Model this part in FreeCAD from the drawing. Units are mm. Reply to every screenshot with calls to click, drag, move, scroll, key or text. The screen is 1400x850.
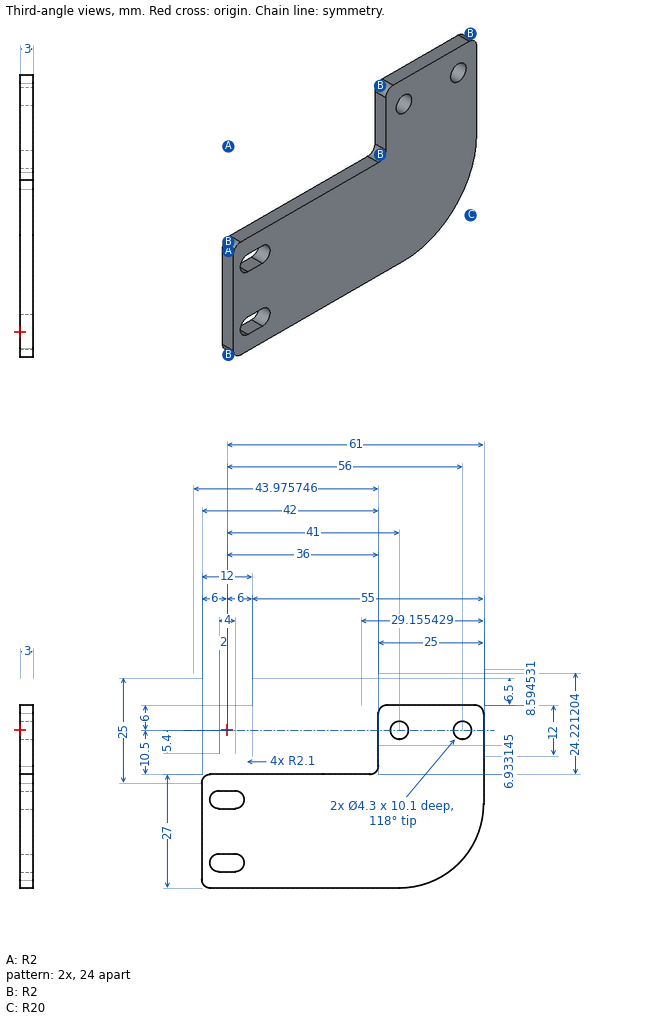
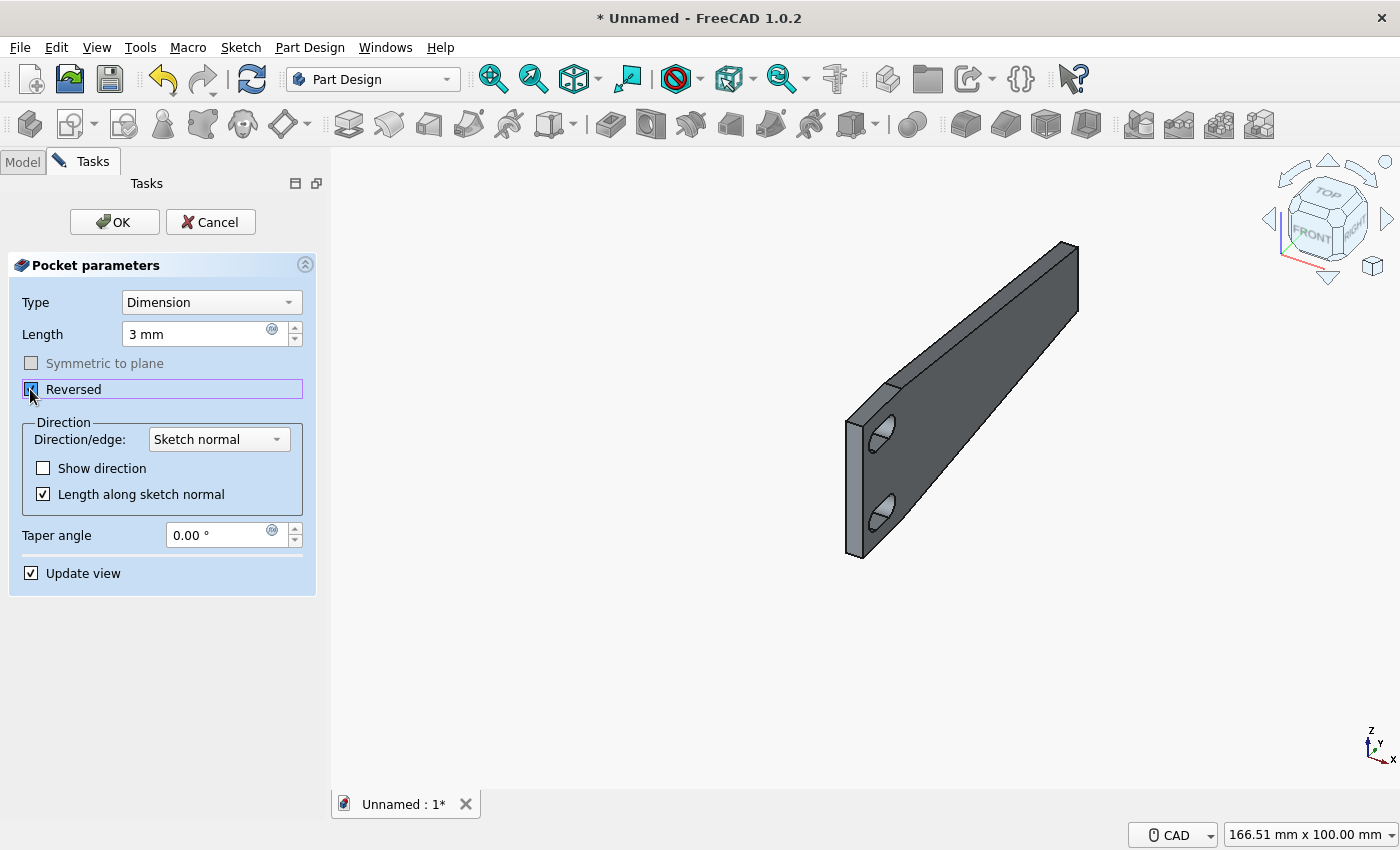
click(115, 222)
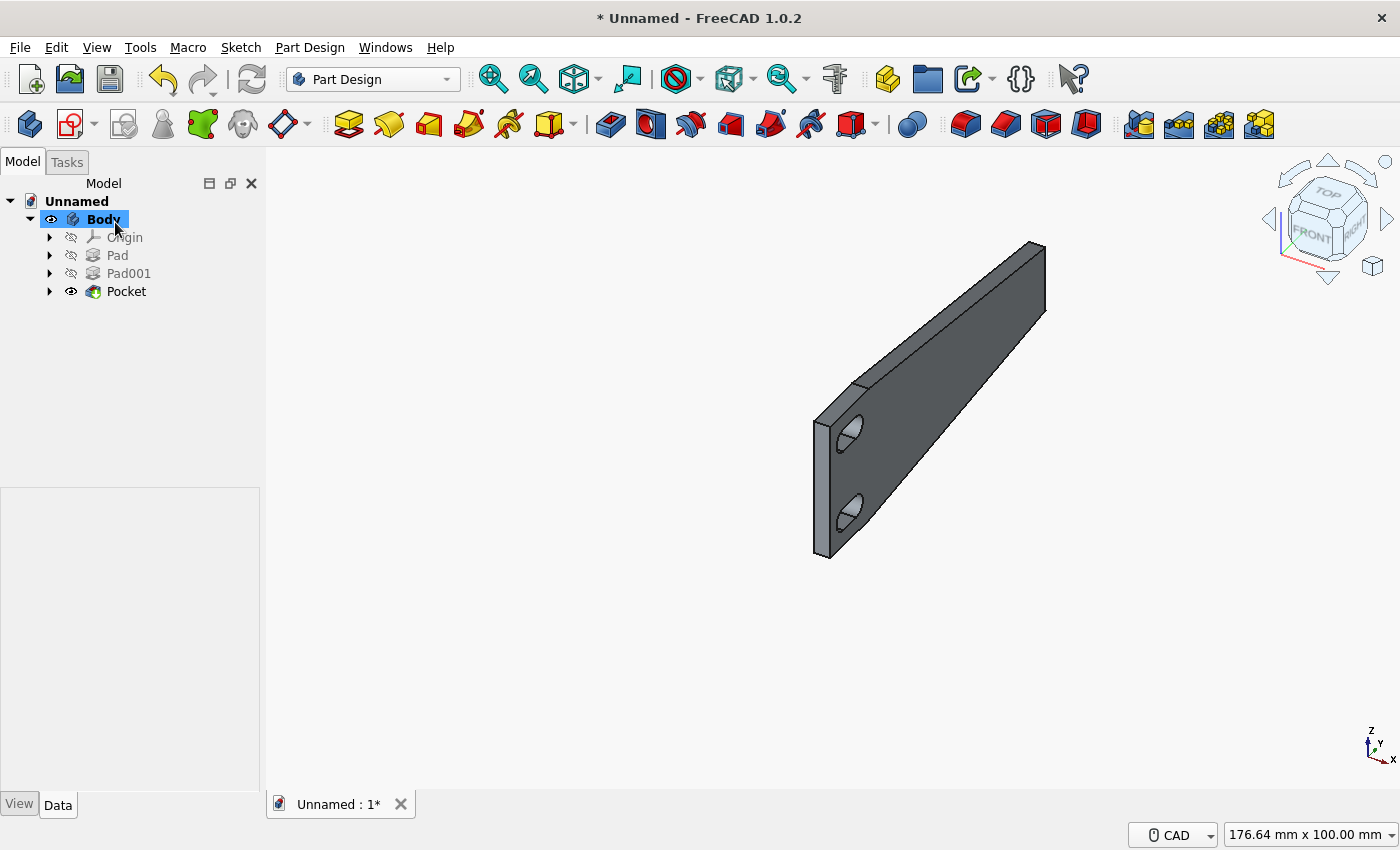
click(822, 423)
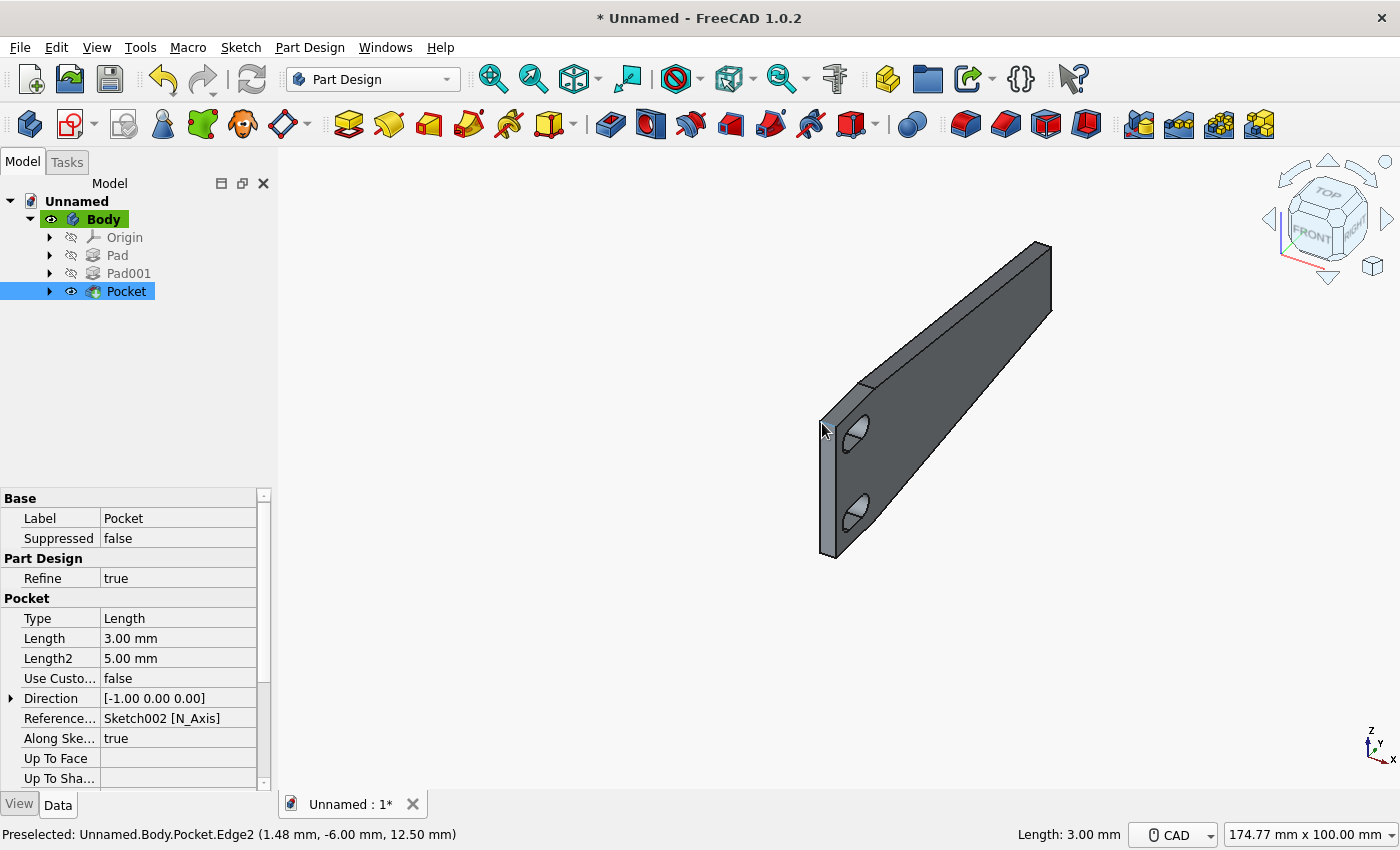
scroll(828, 555, up, 4)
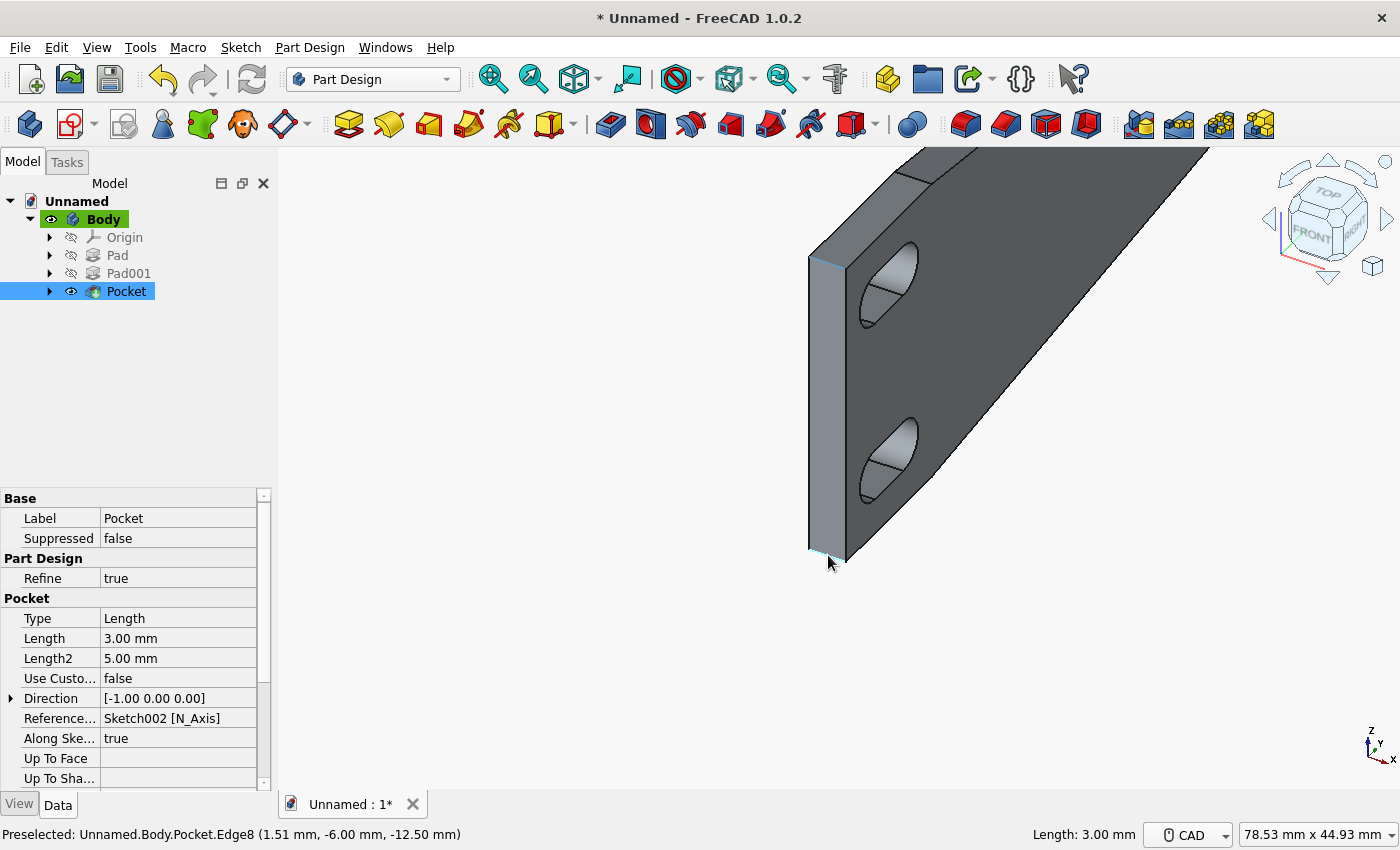
click(494, 80)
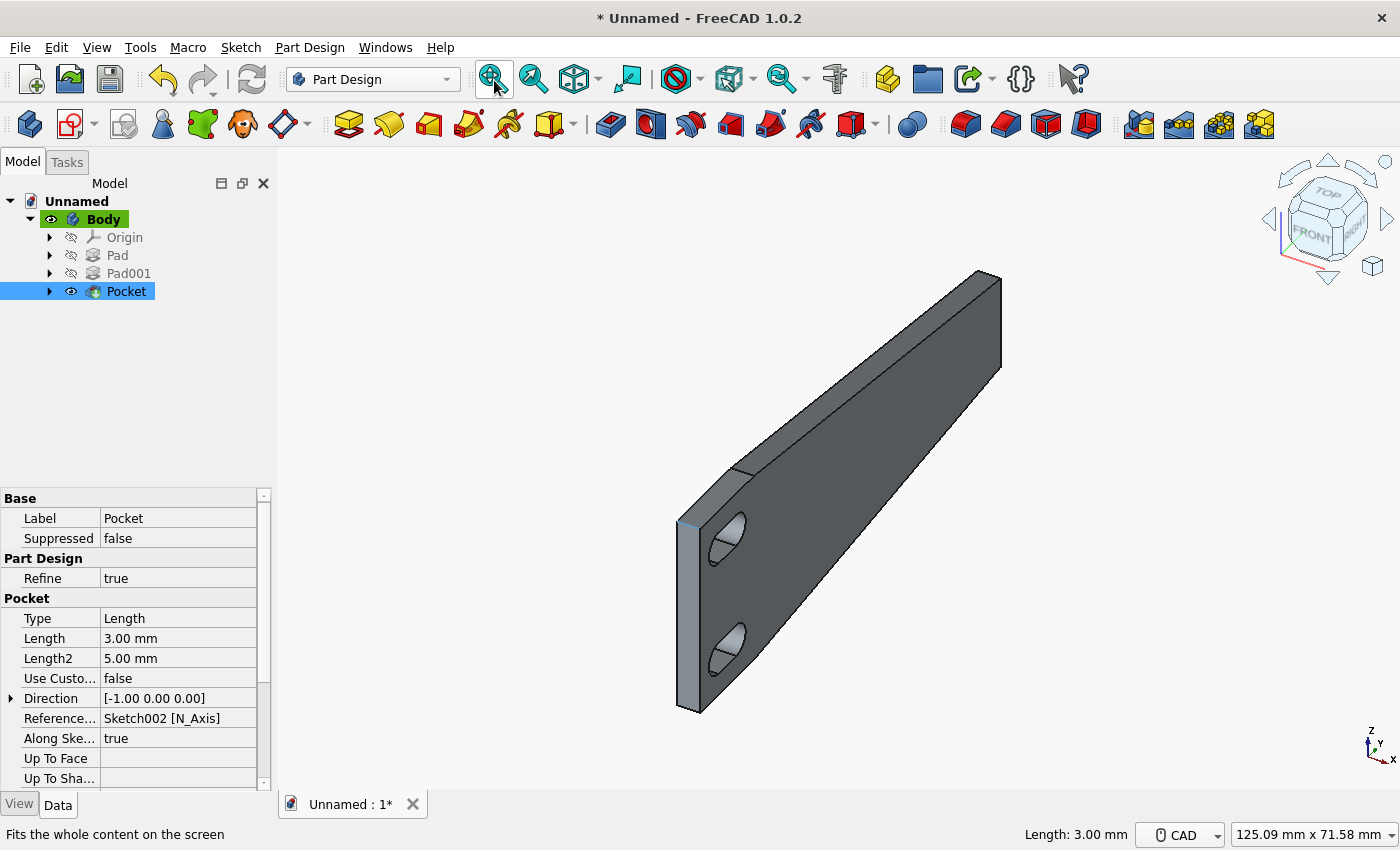
key(0)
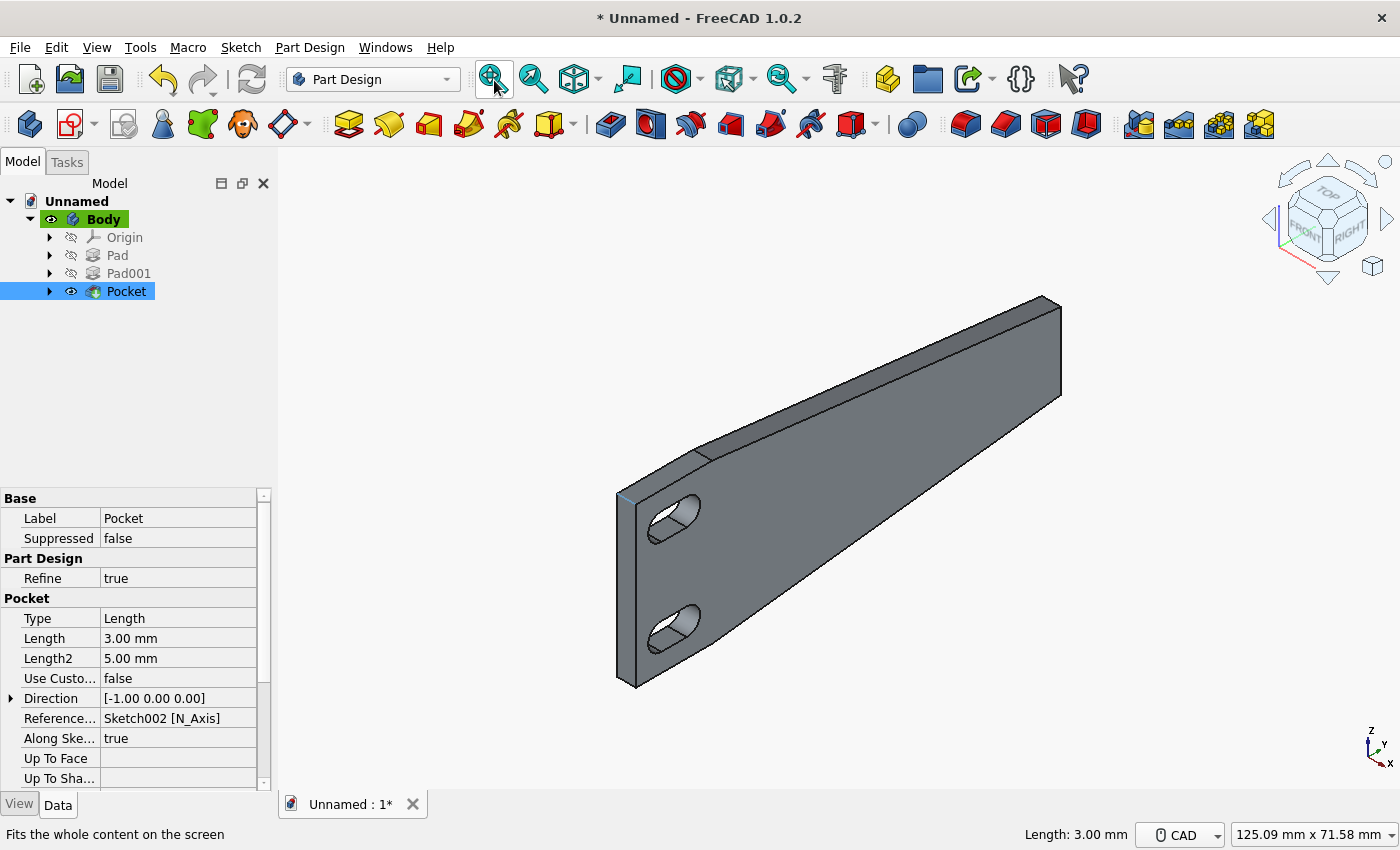
key(2)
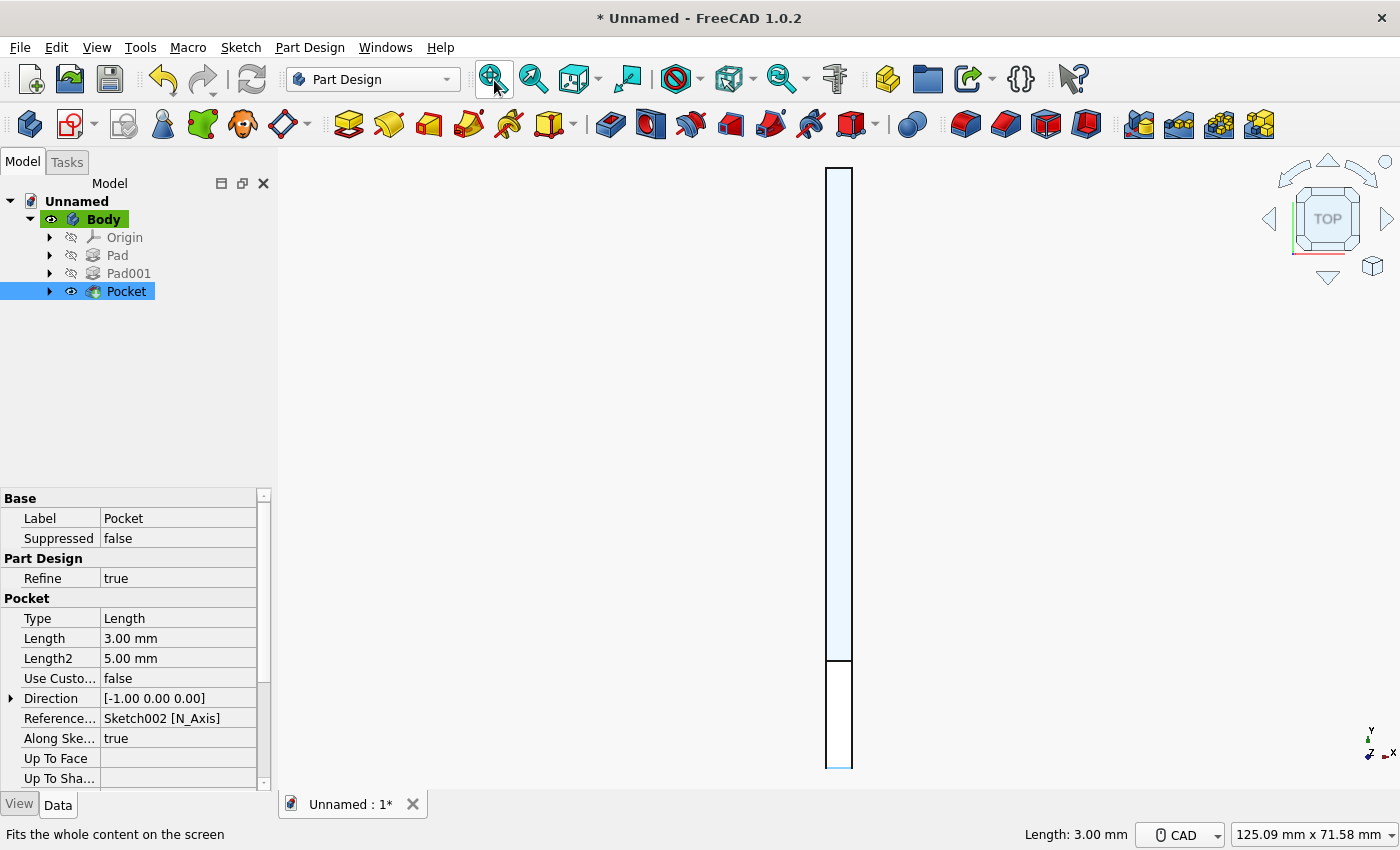
key(1)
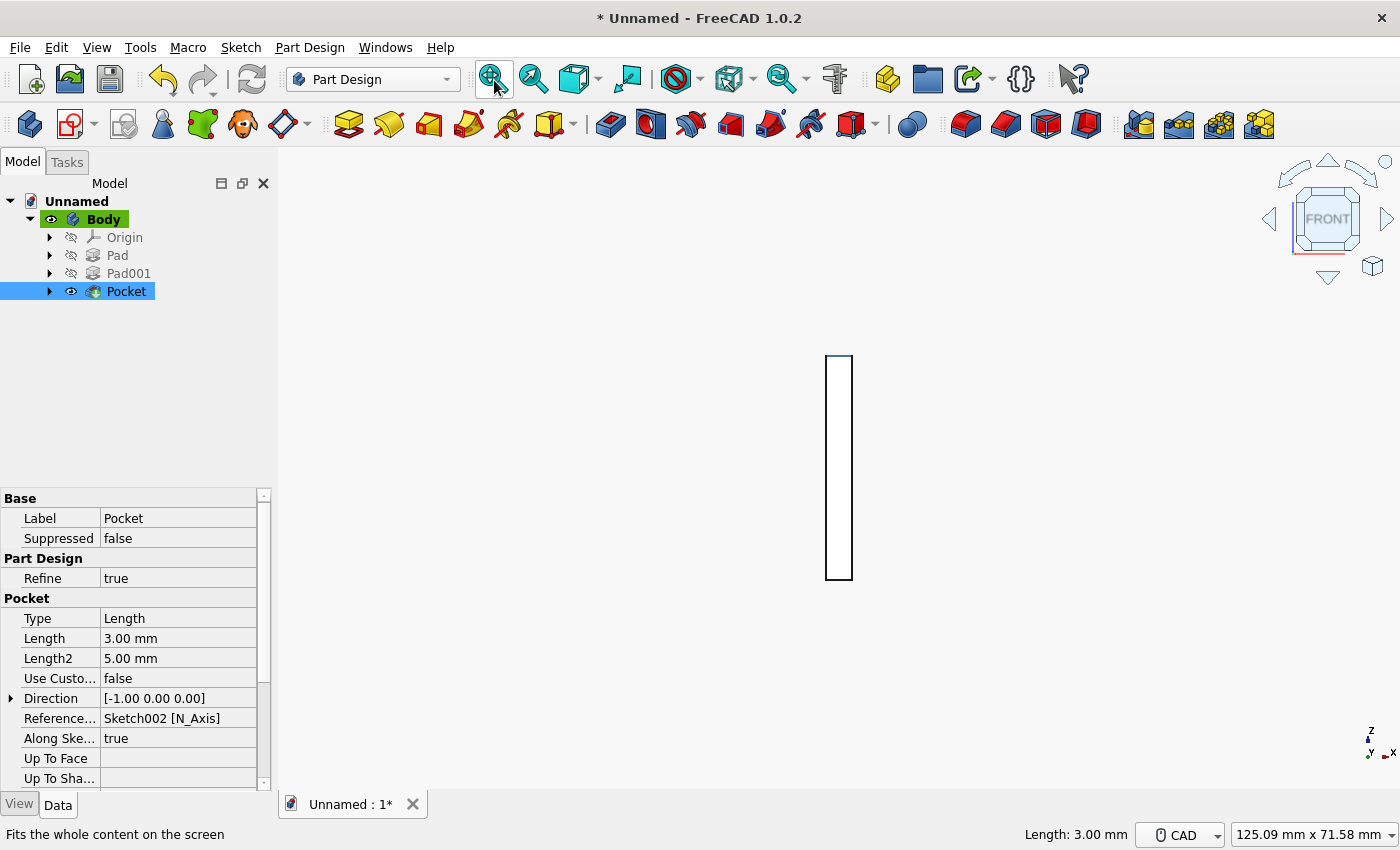
click(494, 80)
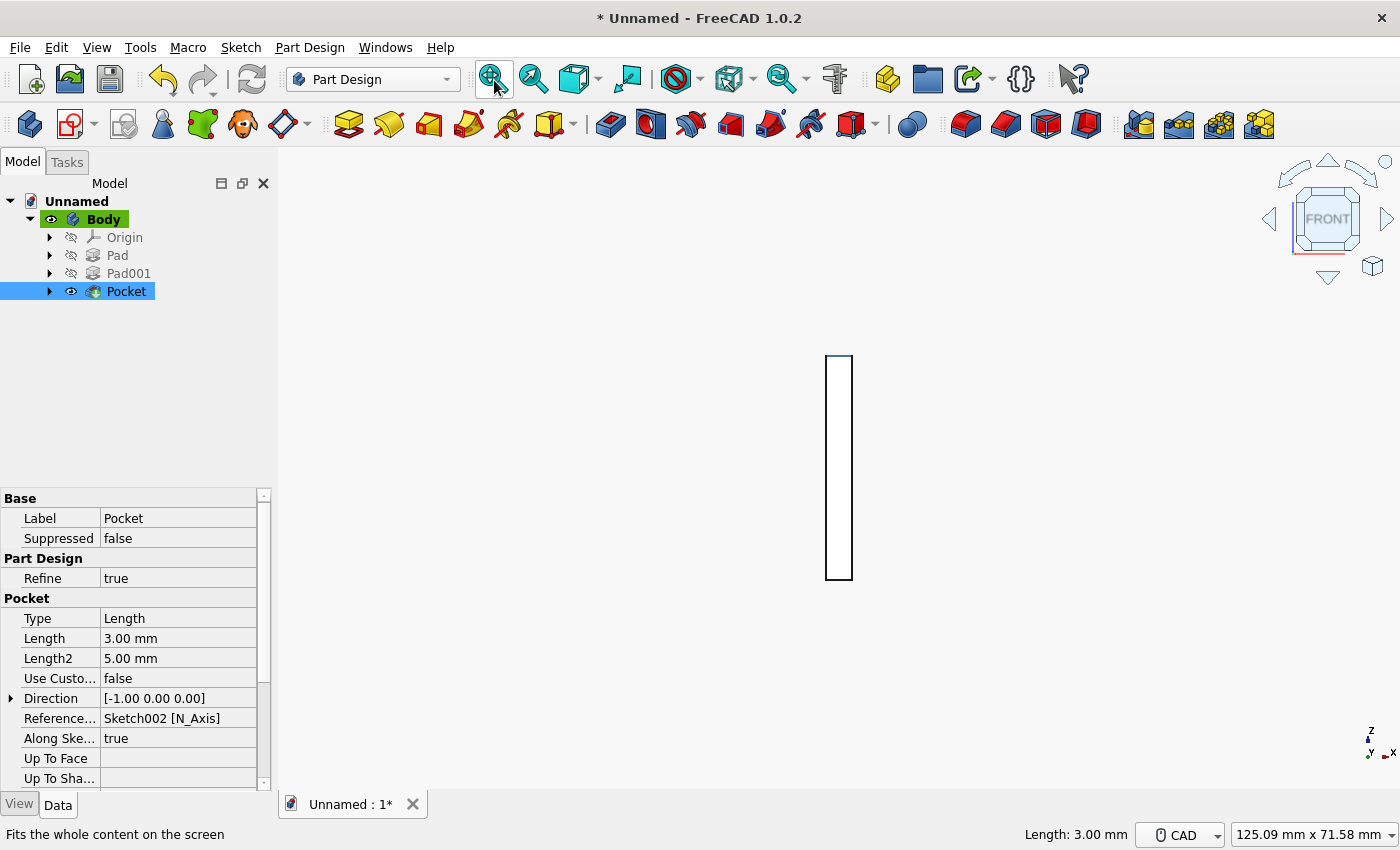
click(839, 579, ctrl)